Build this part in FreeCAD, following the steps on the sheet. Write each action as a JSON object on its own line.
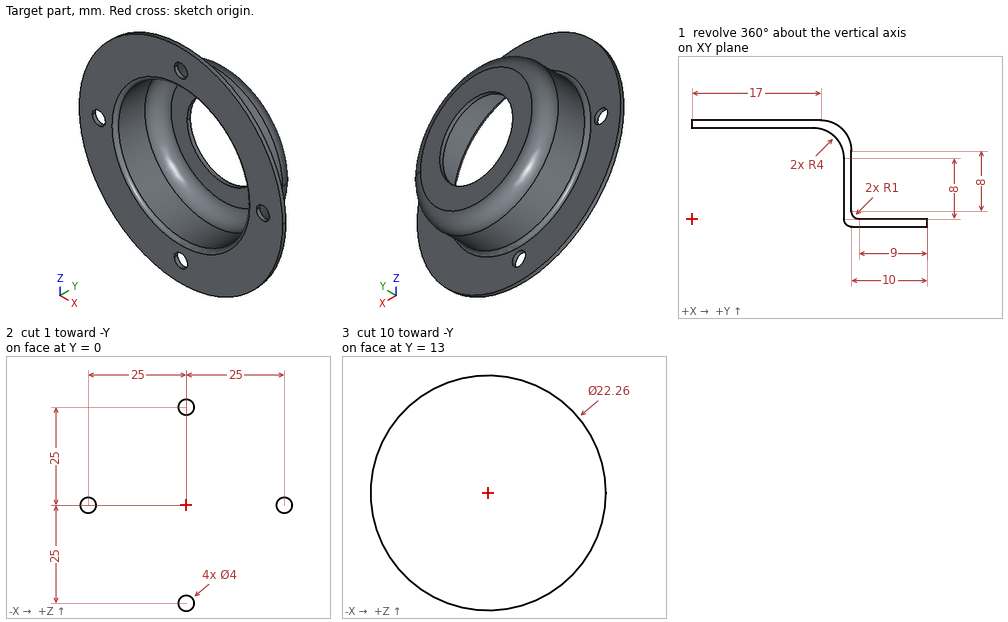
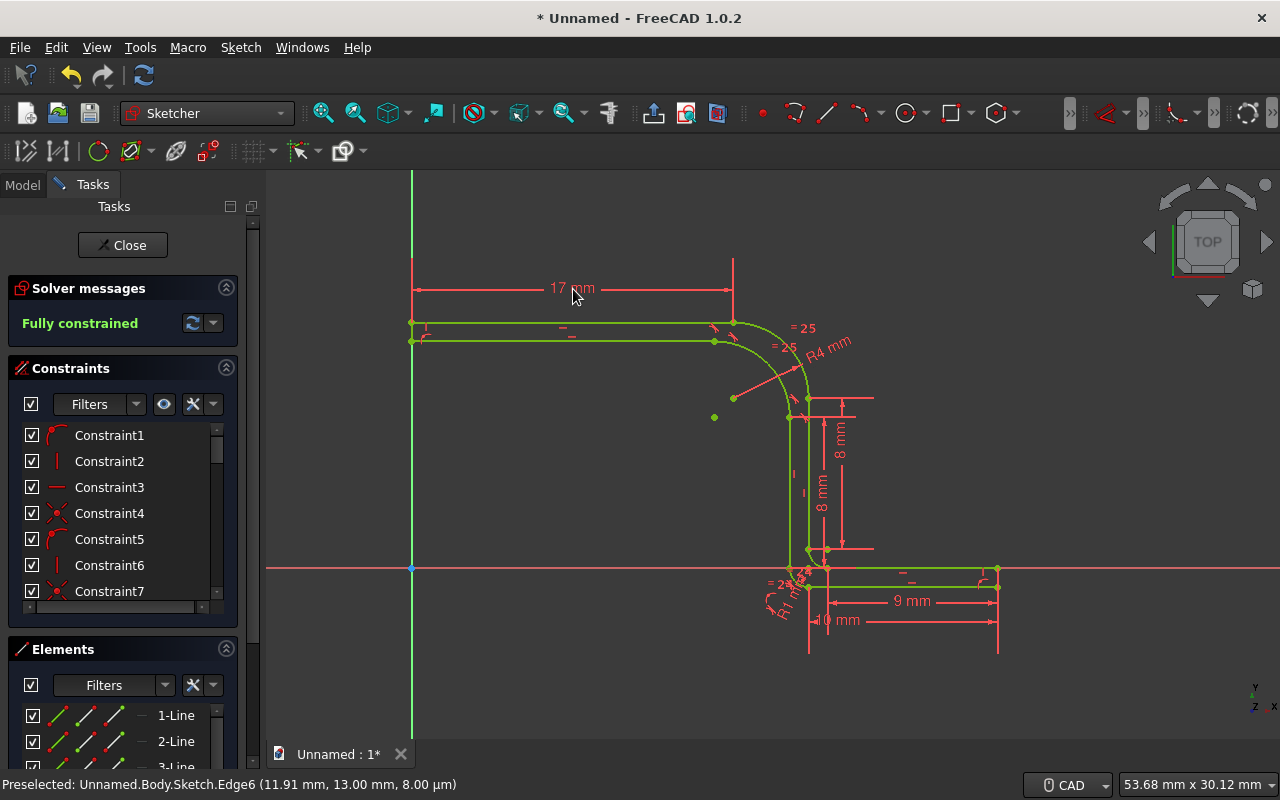
{"action": "left_click", "coordinate": [123, 245]}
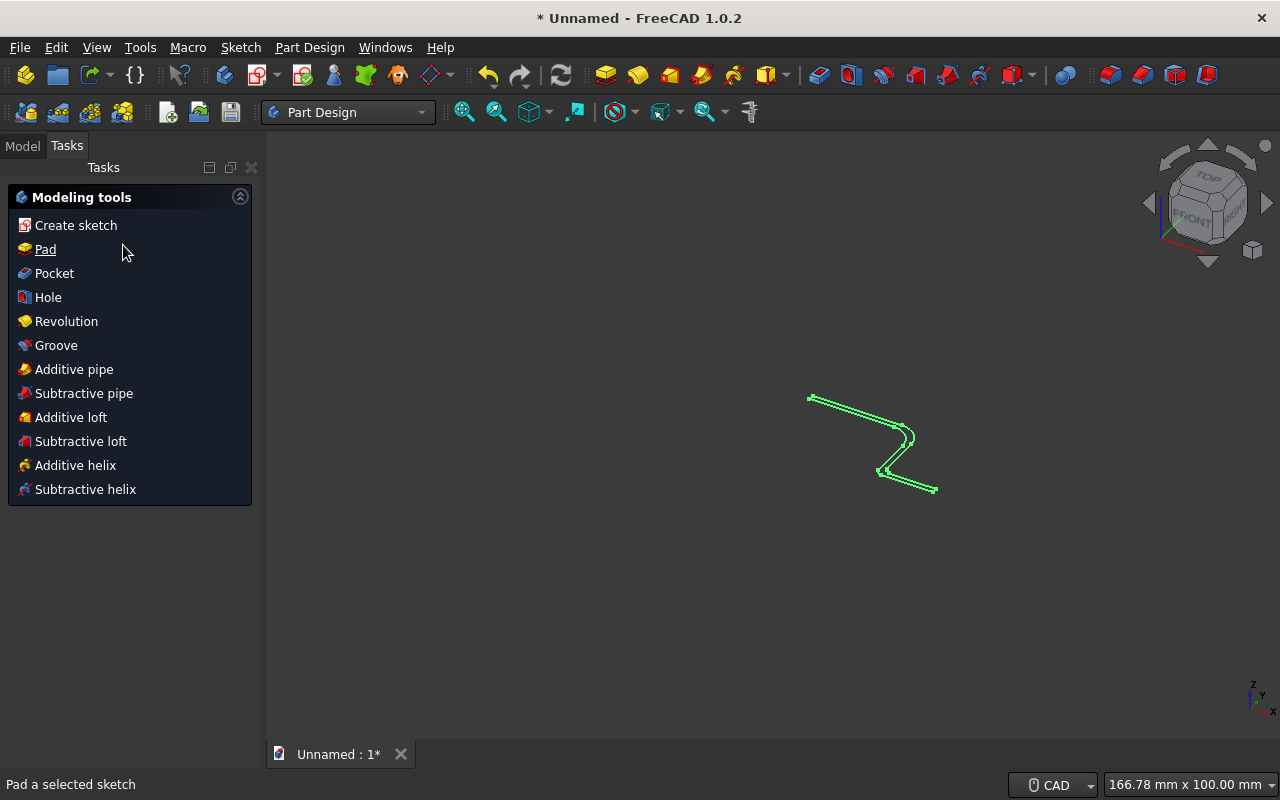
{"action": "left_click", "coordinate": [638, 76]}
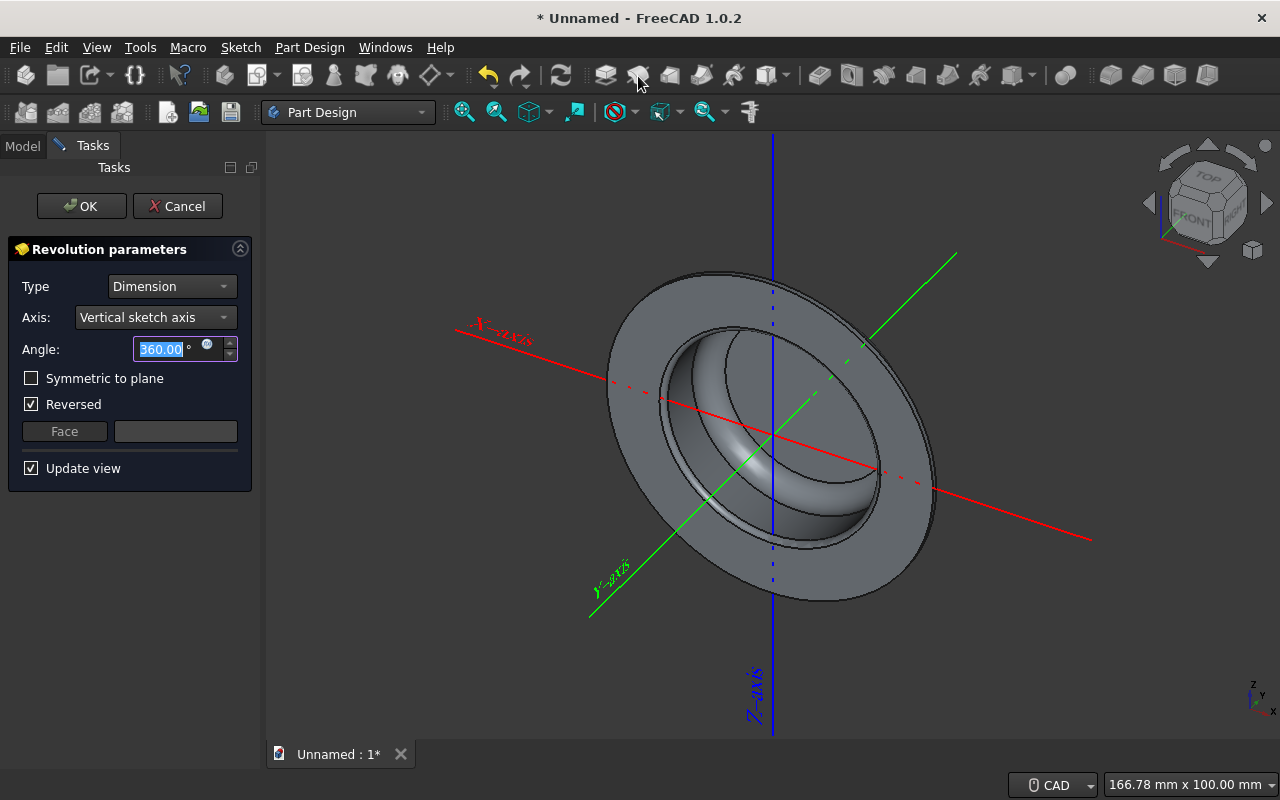
{"action": "left_click", "coordinate": [82, 206]}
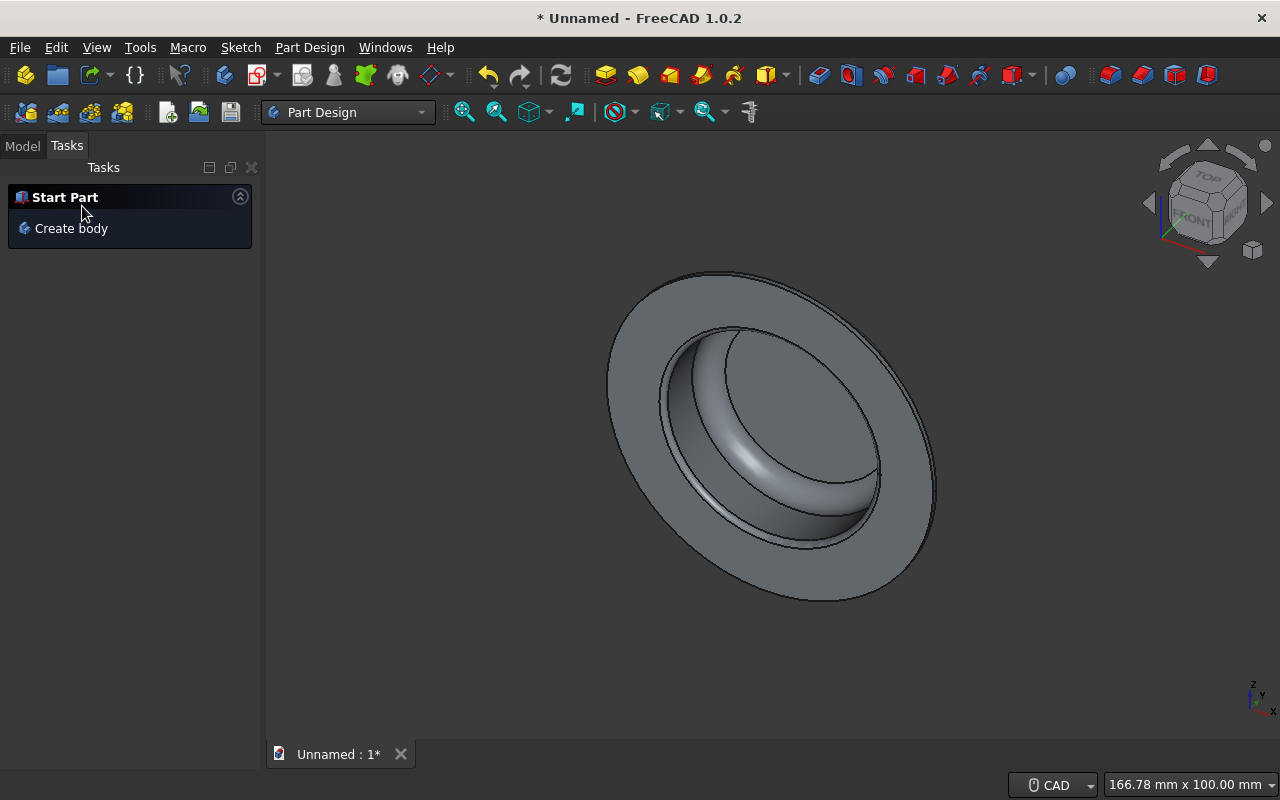
{"action": "key", "text": "4"}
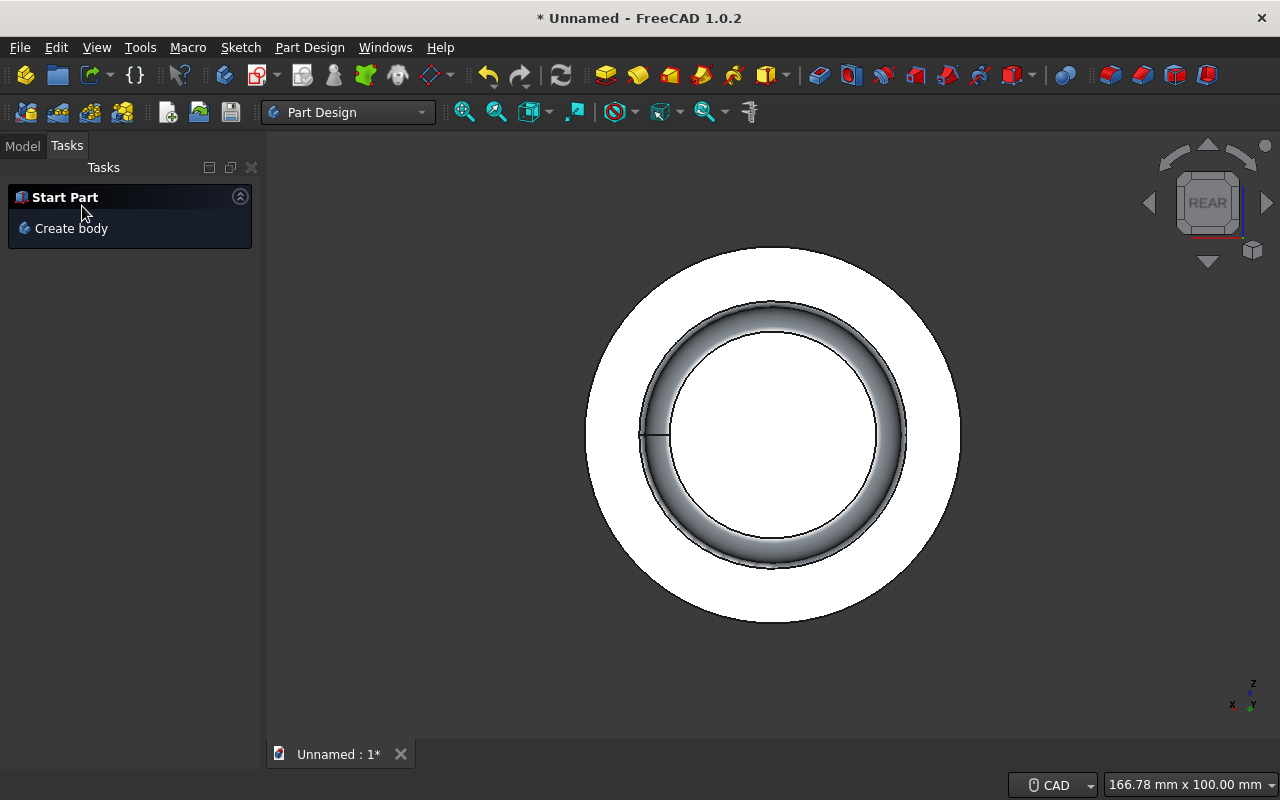
{"action": "left_click", "coordinate": [611, 434]}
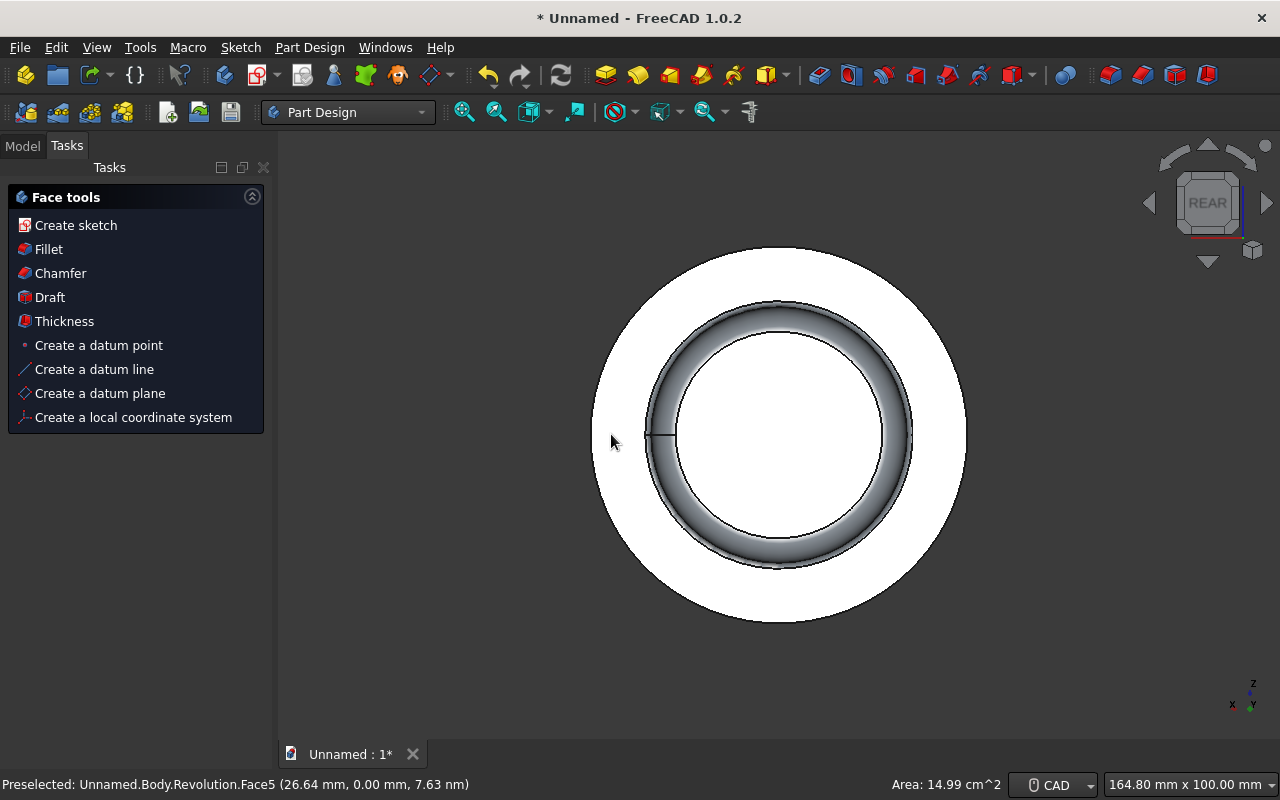
{"action": "left_click", "coordinate": [258, 76]}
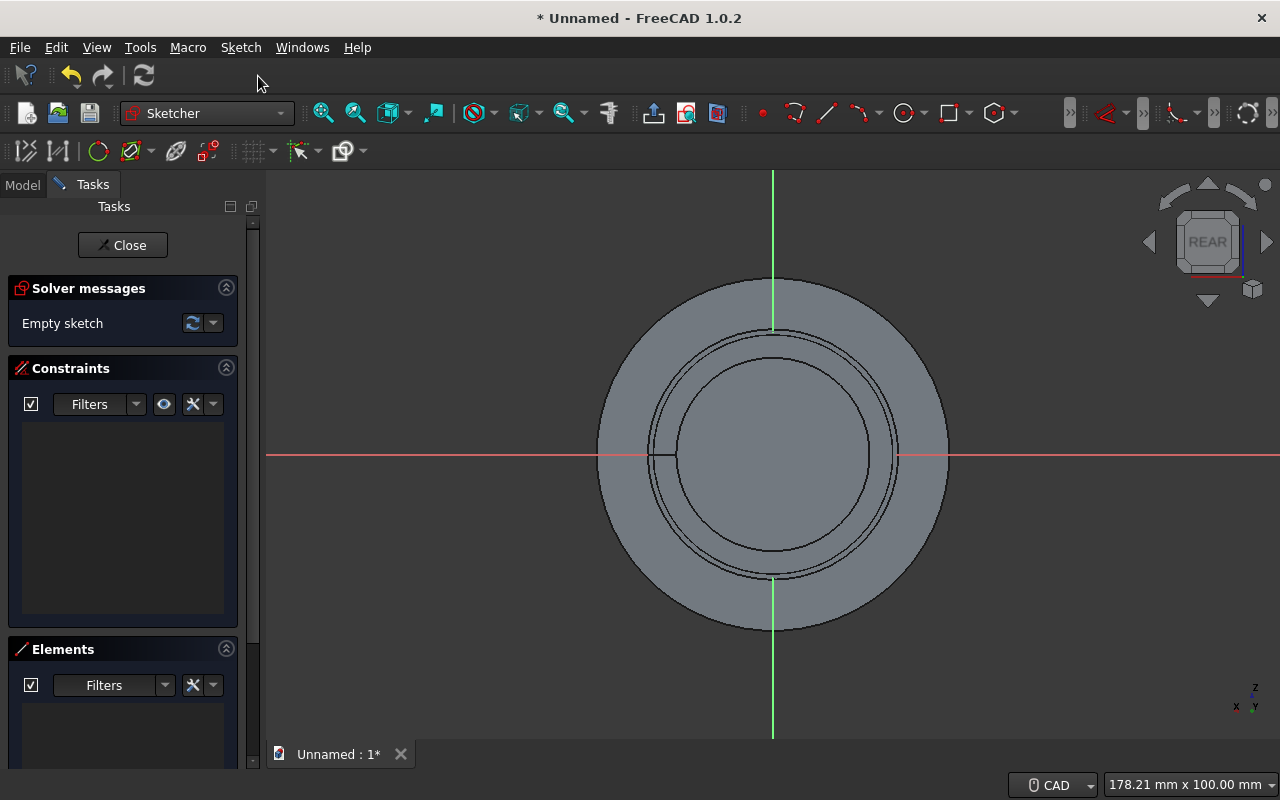
{"action": "left_click", "coordinate": [718, 114]}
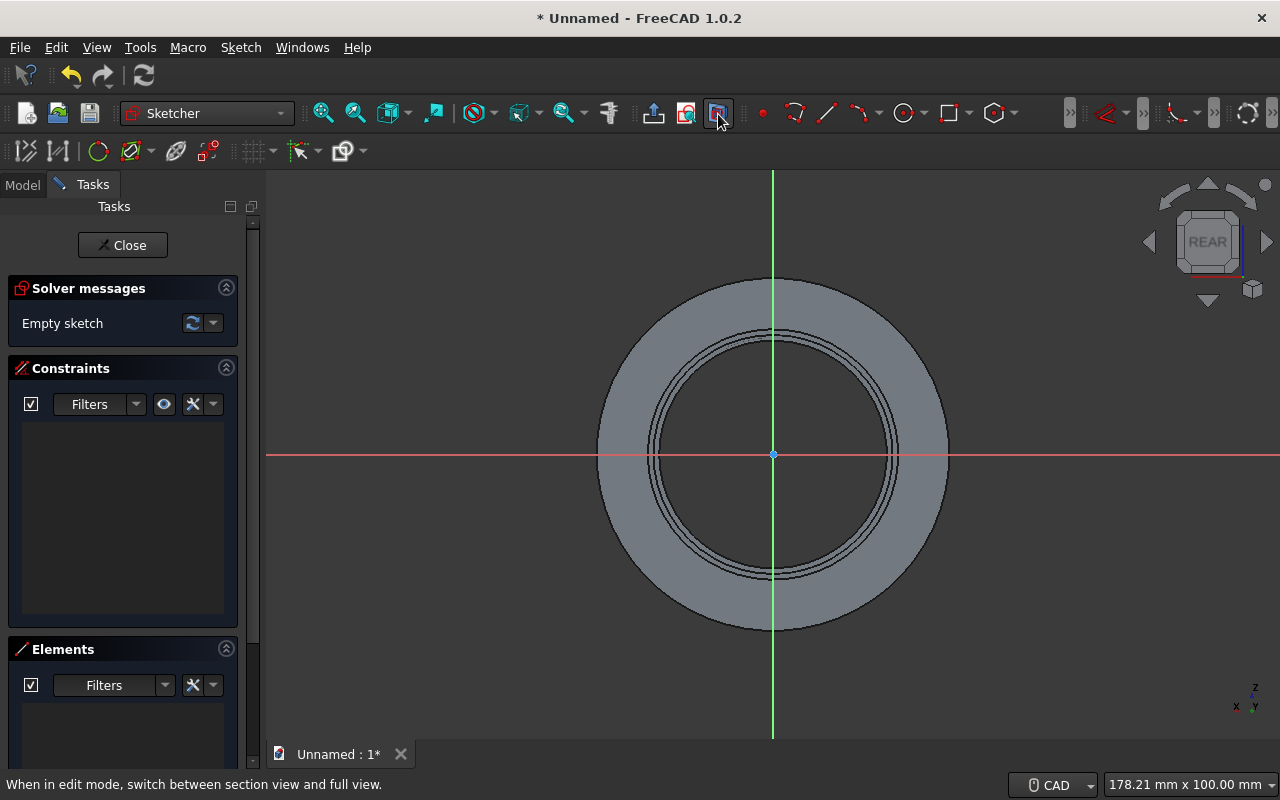
{"action": "left_click", "coordinate": [904, 114]}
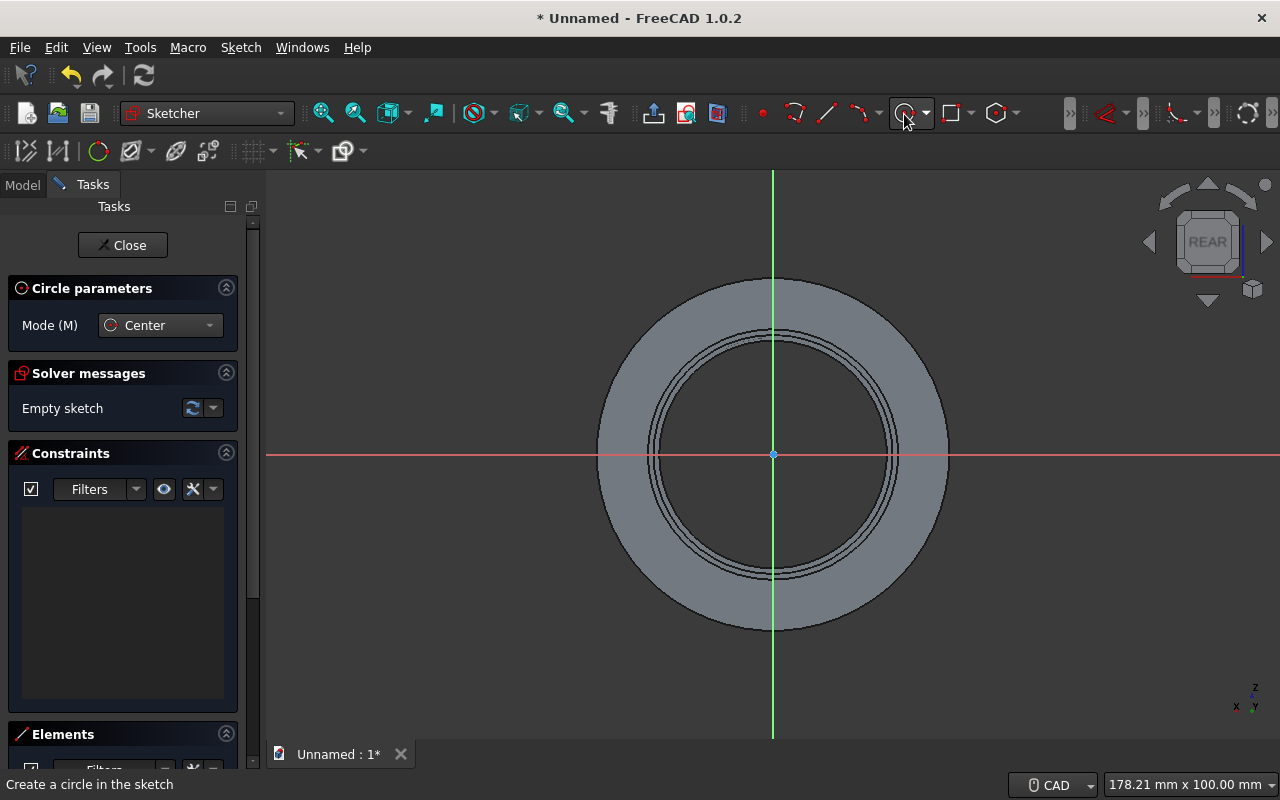
{"action": "scroll", "coordinate": [773, 597], "scroll_direction": "up", "scroll_amount": 4}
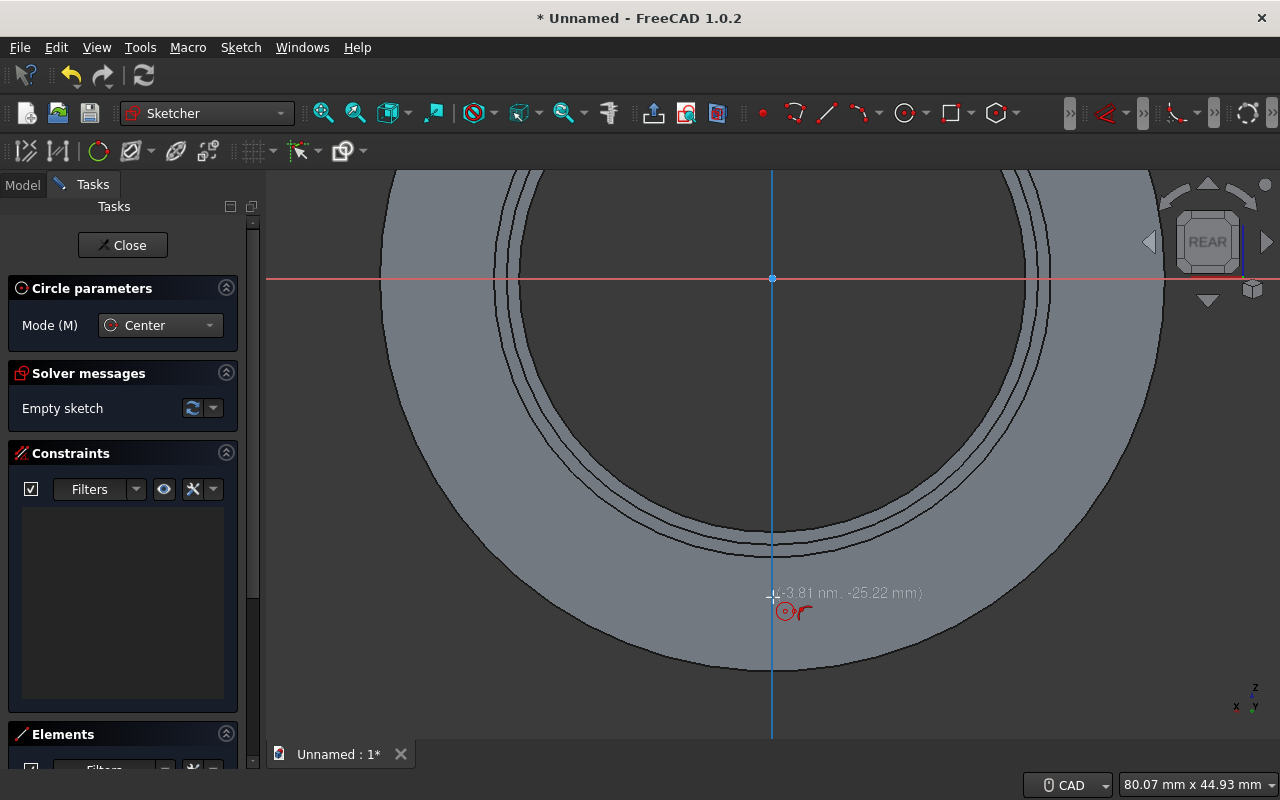
{"action": "left_click", "coordinate": [772, 596]}
{"action": "left_click", "coordinate": [790, 578]}